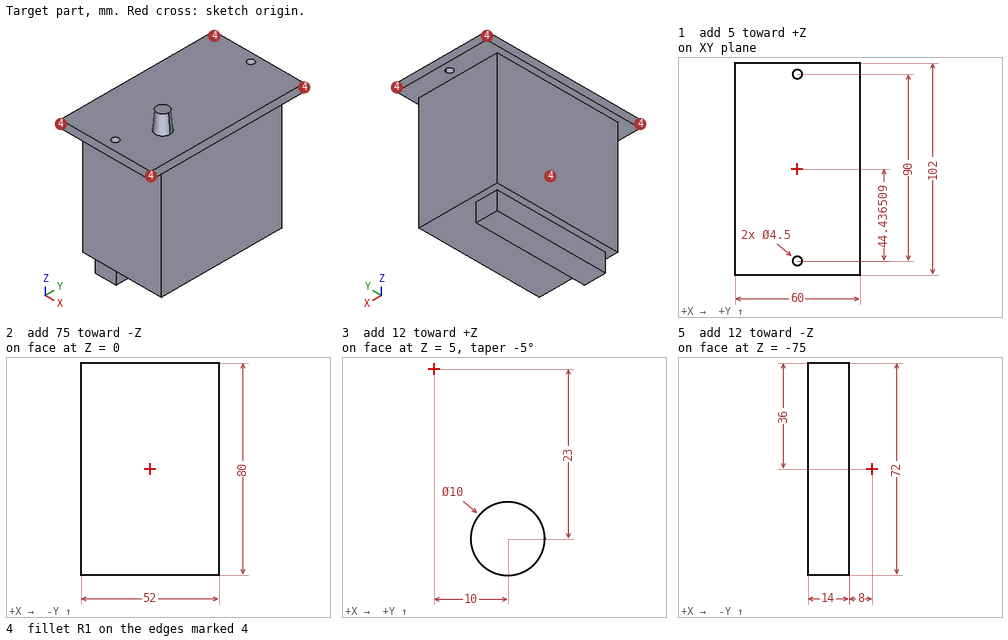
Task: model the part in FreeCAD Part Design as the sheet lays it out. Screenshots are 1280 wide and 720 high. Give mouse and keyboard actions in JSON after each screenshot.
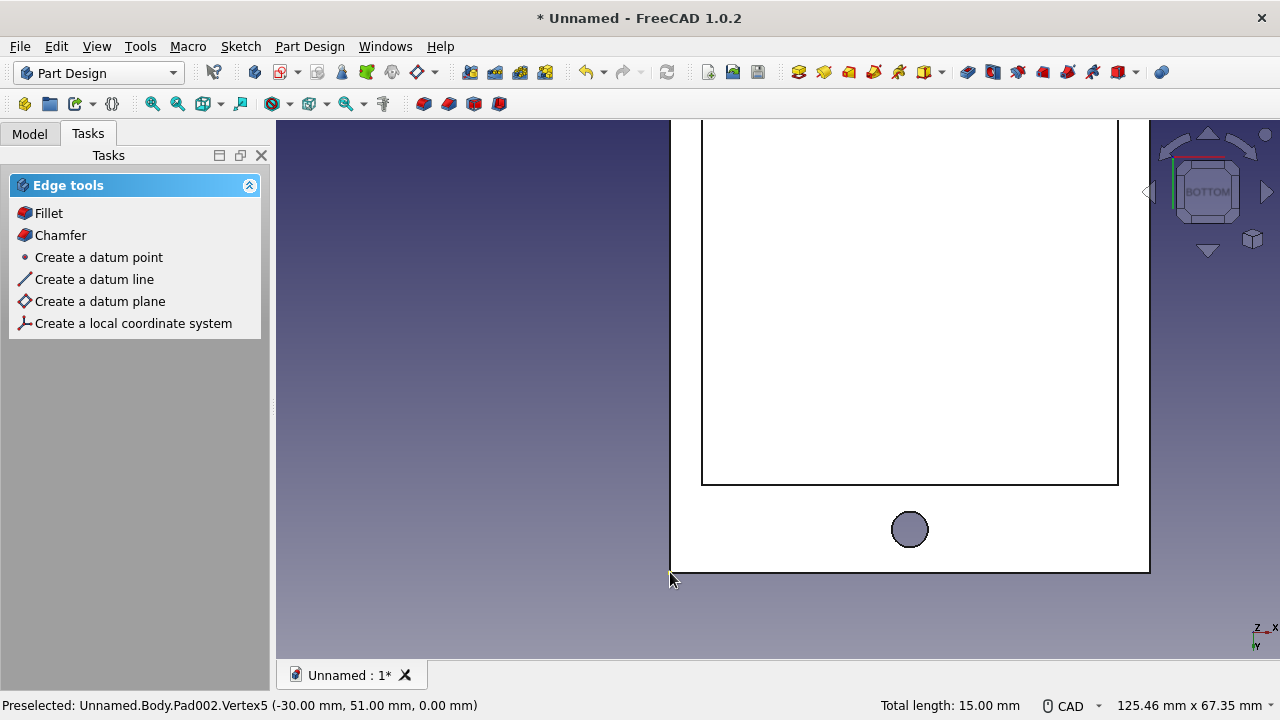
{"action": "left_click", "coordinate": [153, 104]}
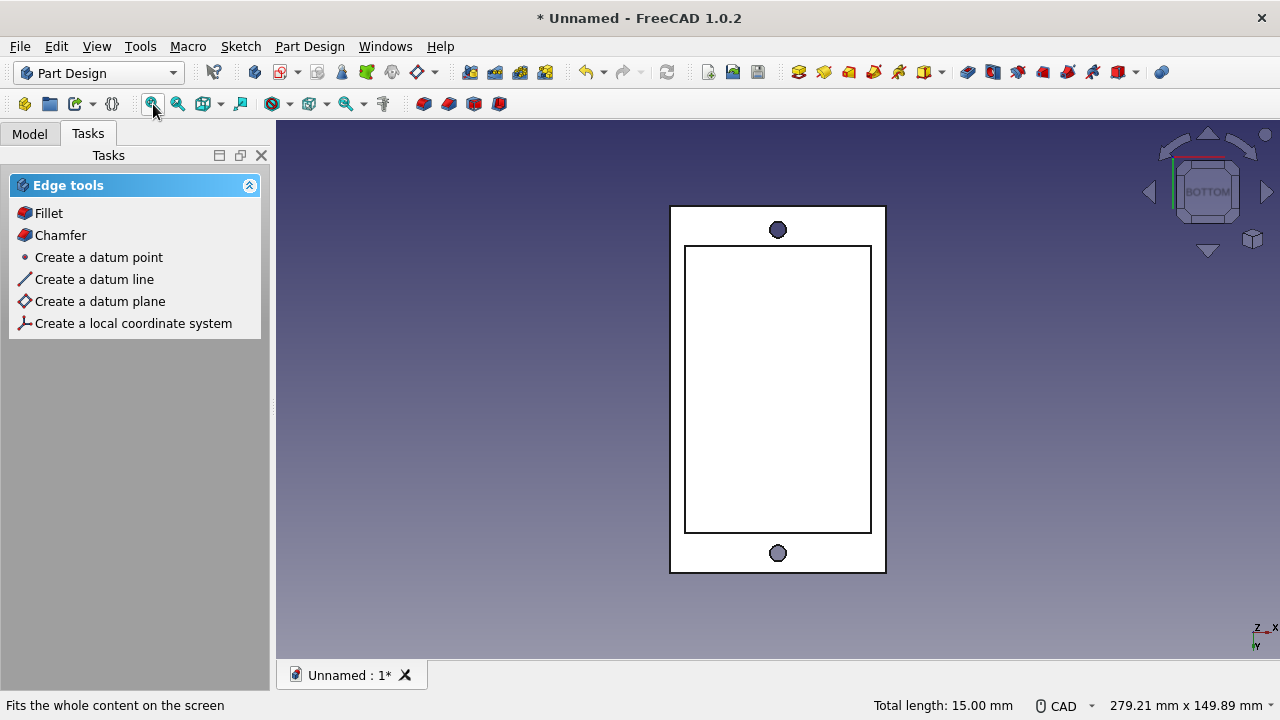
{"action": "key", "text": "4"}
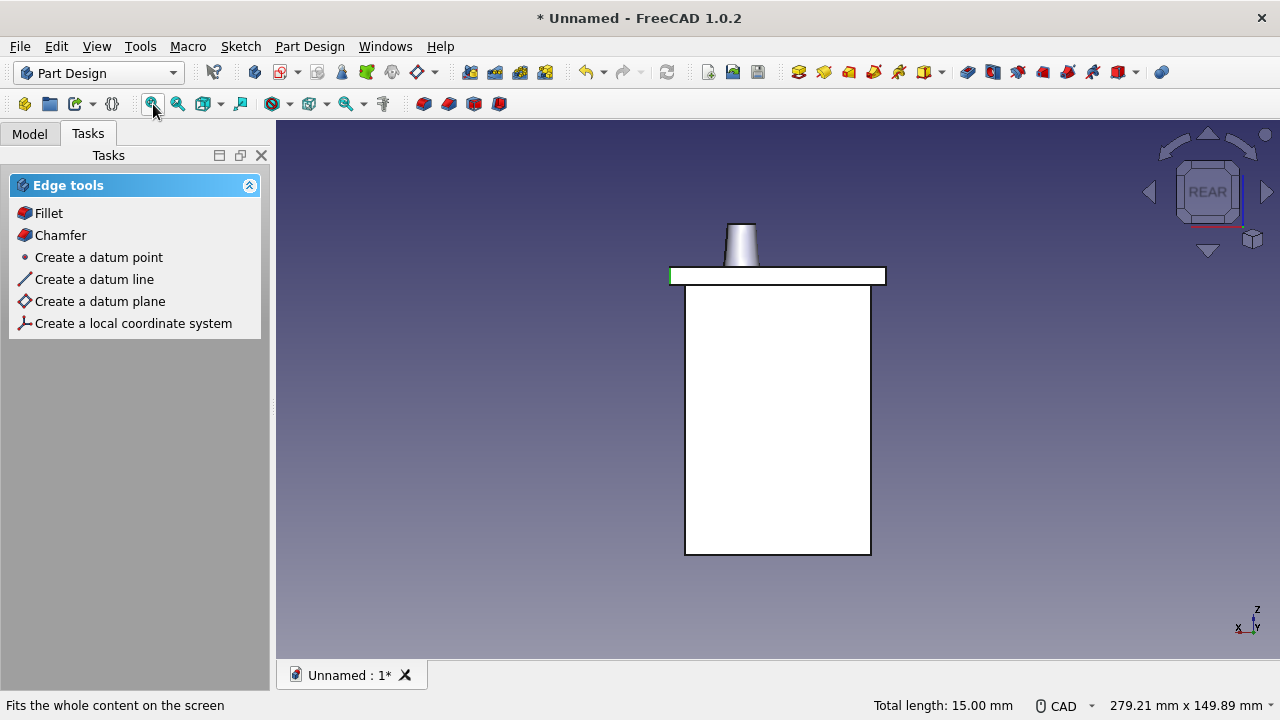
{"action": "left_click", "coordinate": [886, 275], "text": "ctrl"}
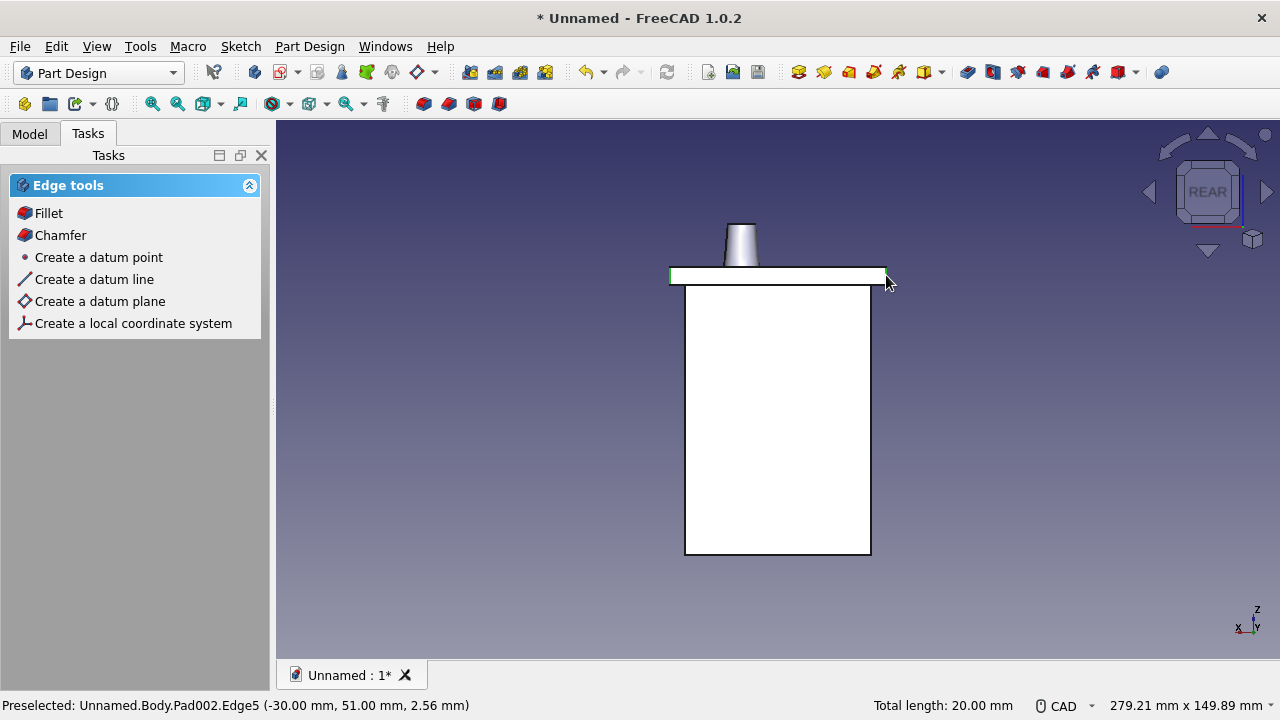
{"action": "left_click", "coordinate": [424, 104]}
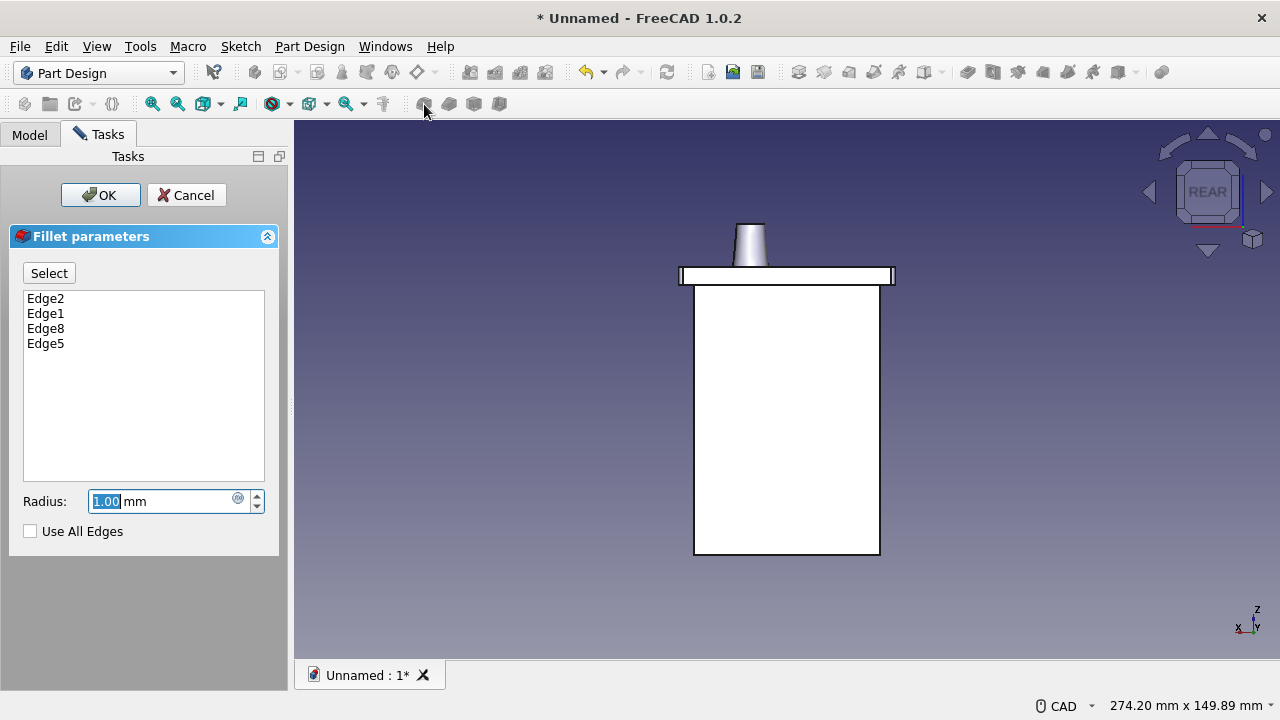
{"action": "type", "text": "1"}
{"action": "key", "text": "Tab"}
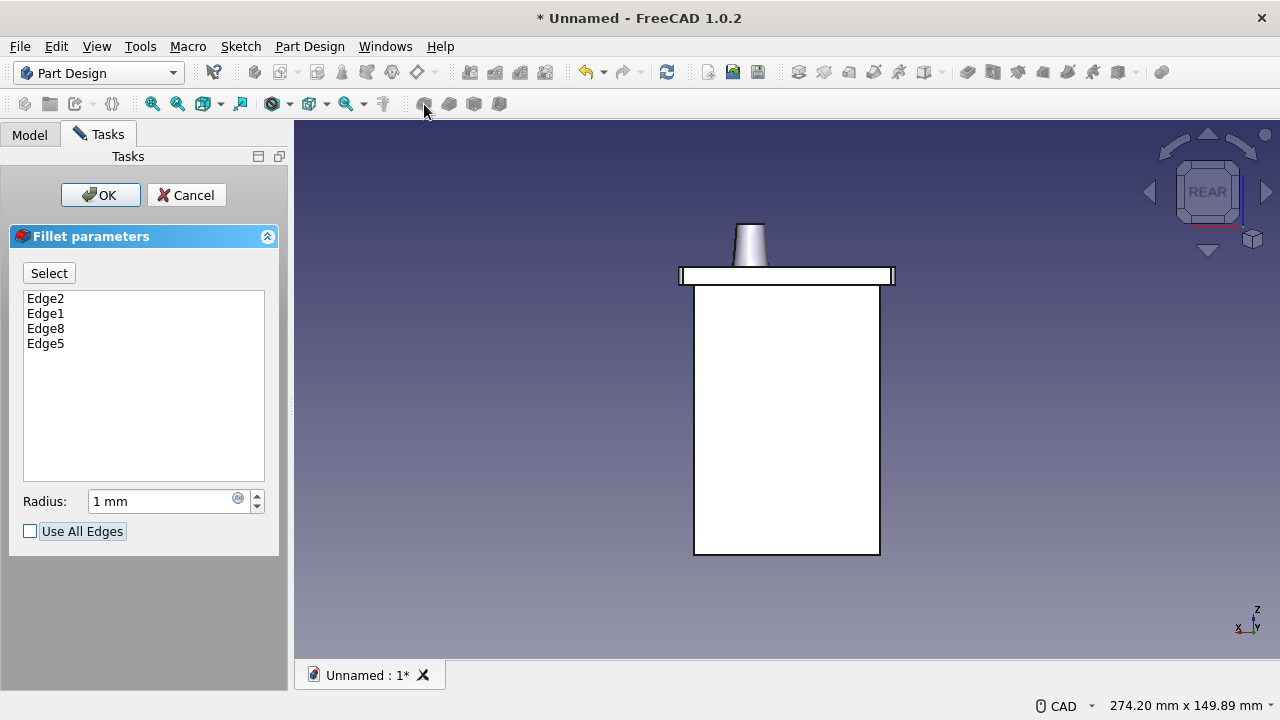
{"action": "left_click", "coordinate": [101, 195]}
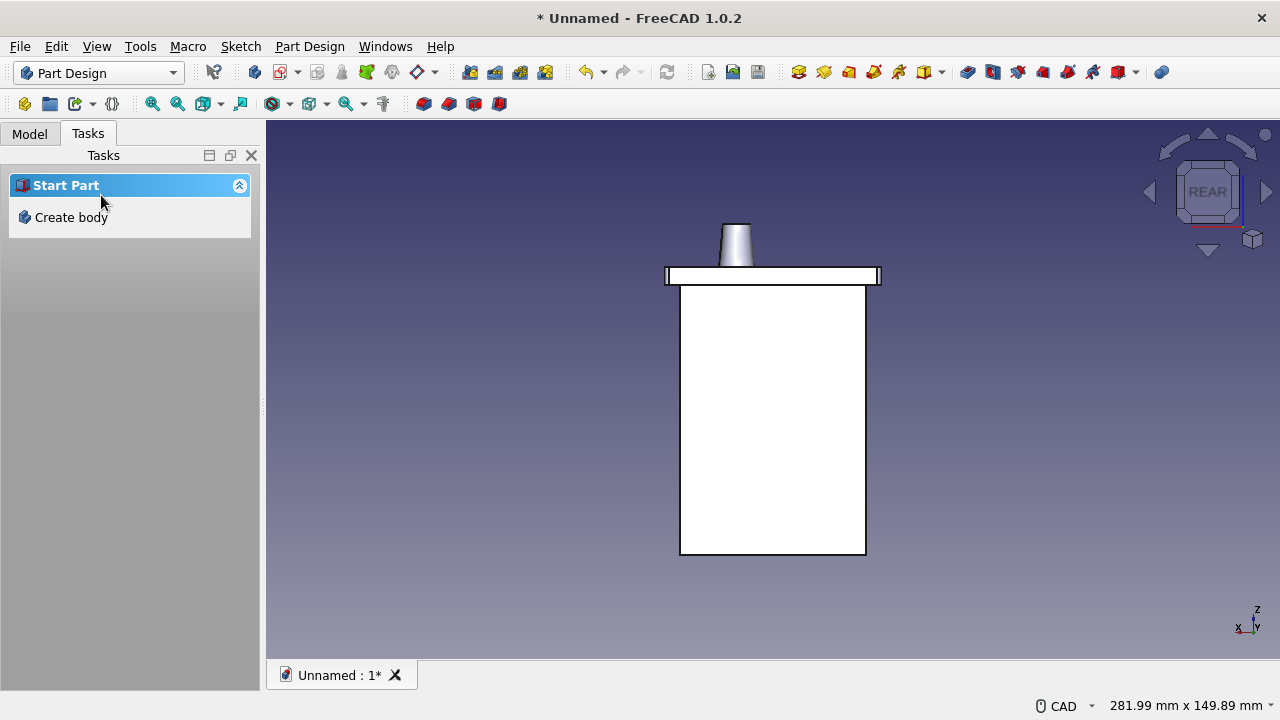
{"action": "key", "text": "5"}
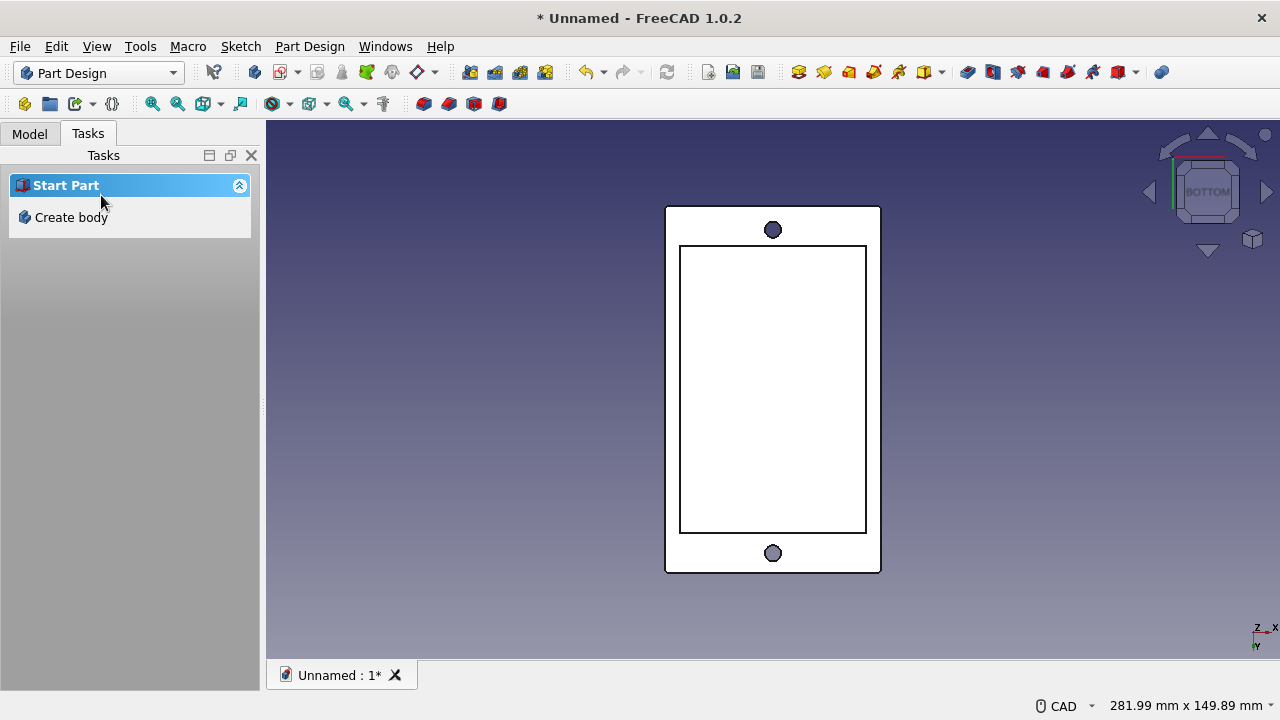
{"action": "left_click", "coordinate": [773, 430]}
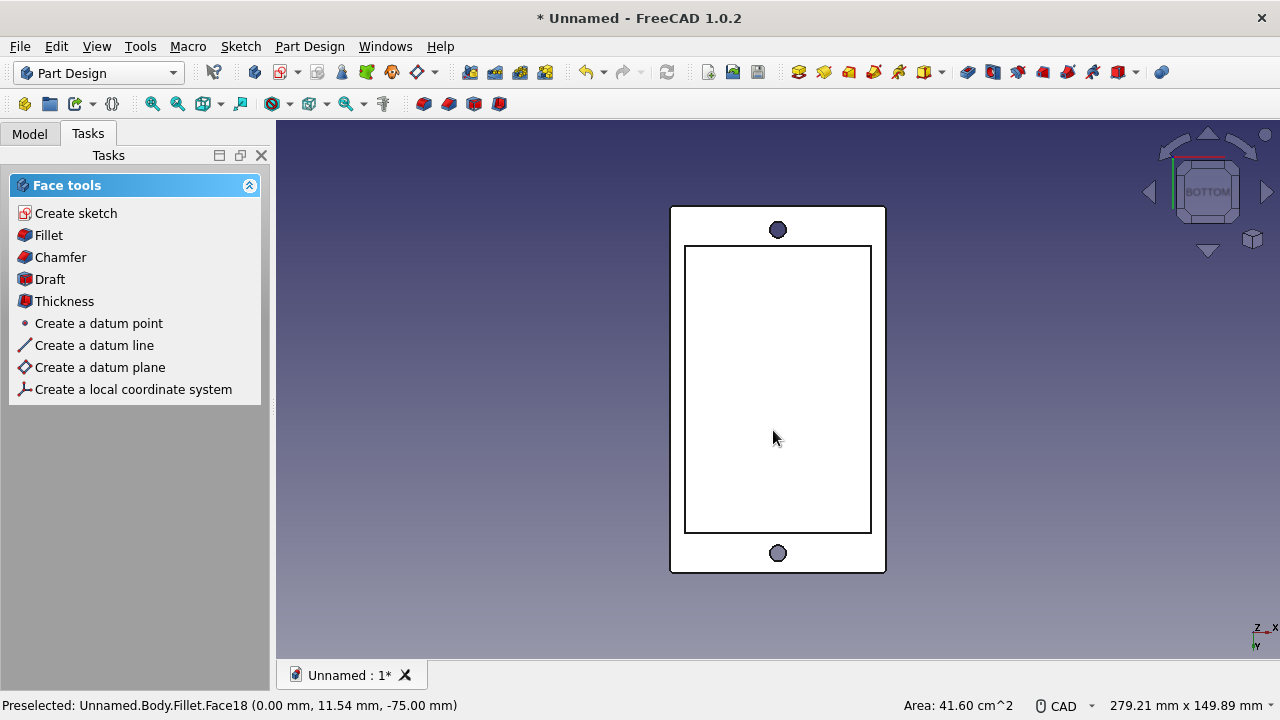
{"action": "left_click", "coordinate": [280, 72]}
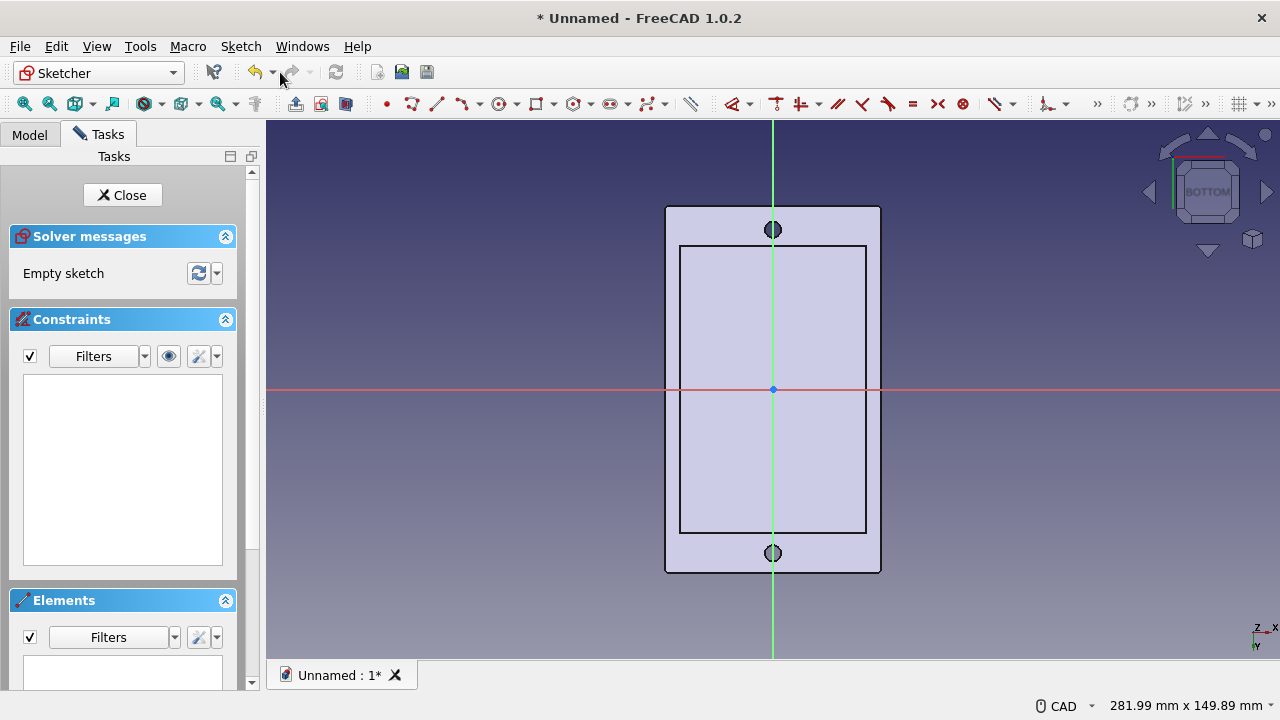
{"action": "key", "text": "g r"}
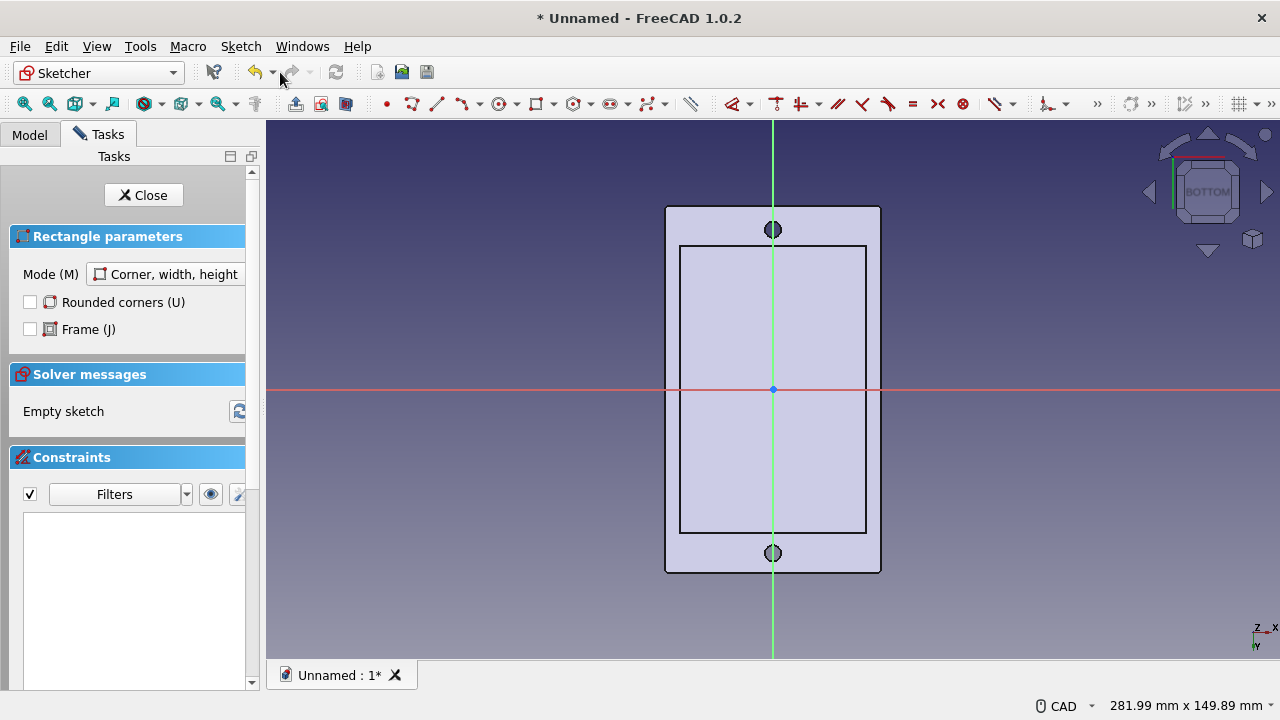
{"action": "left_click", "coordinate": [694, 260]}
{"action": "mouse_move", "coordinate": [744, 519]}